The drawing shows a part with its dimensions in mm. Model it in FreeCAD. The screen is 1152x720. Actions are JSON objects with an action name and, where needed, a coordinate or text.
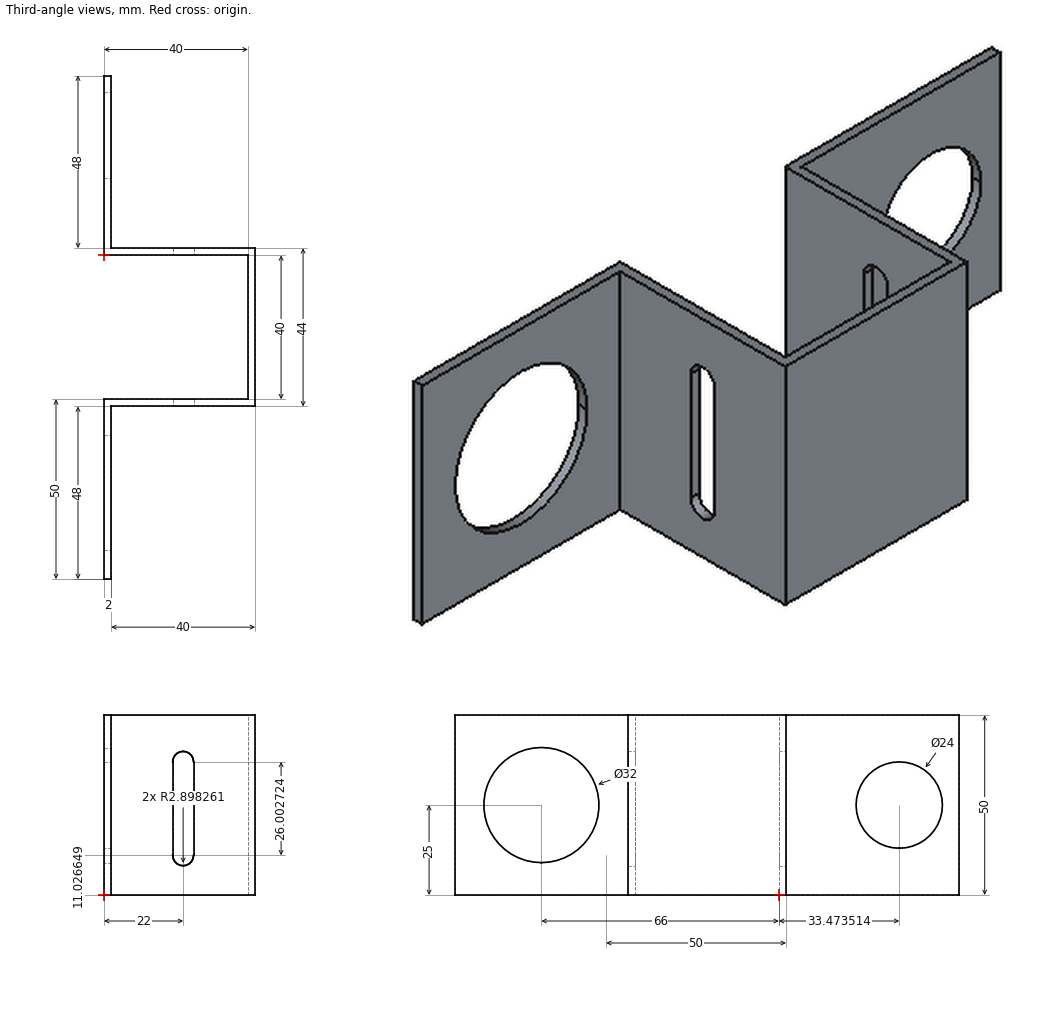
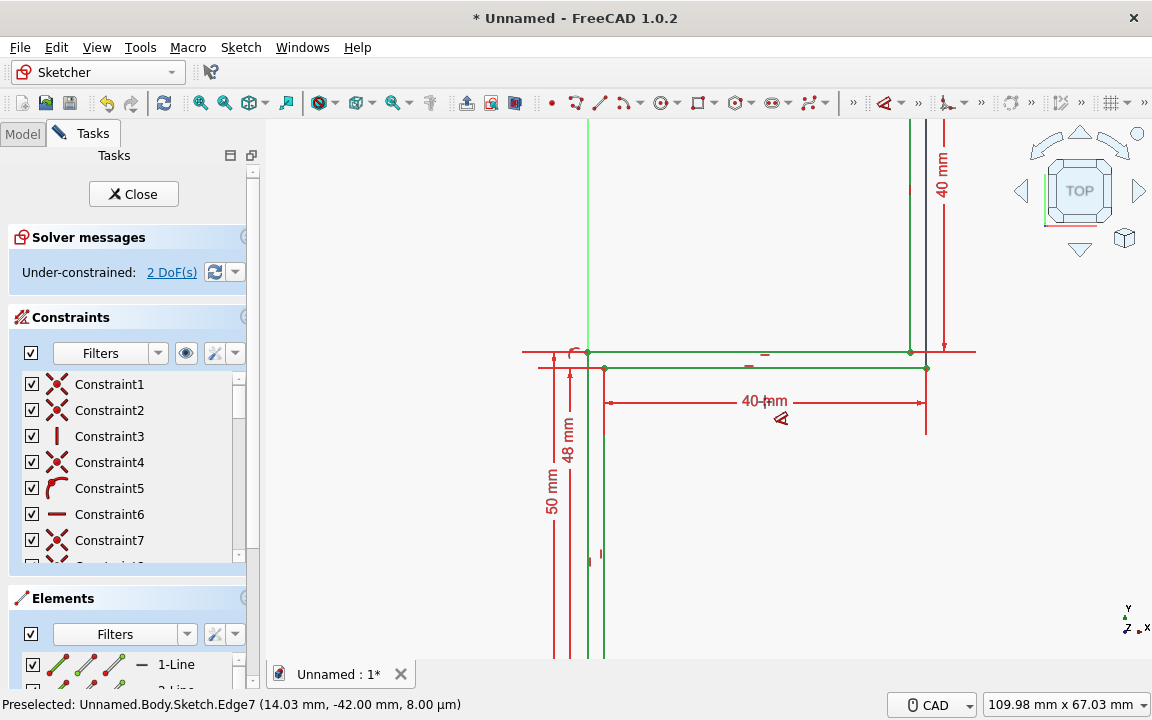
{"action": "left_click", "coordinate": [926, 262]}
{"action": "left_click", "coordinate": [960, 258]}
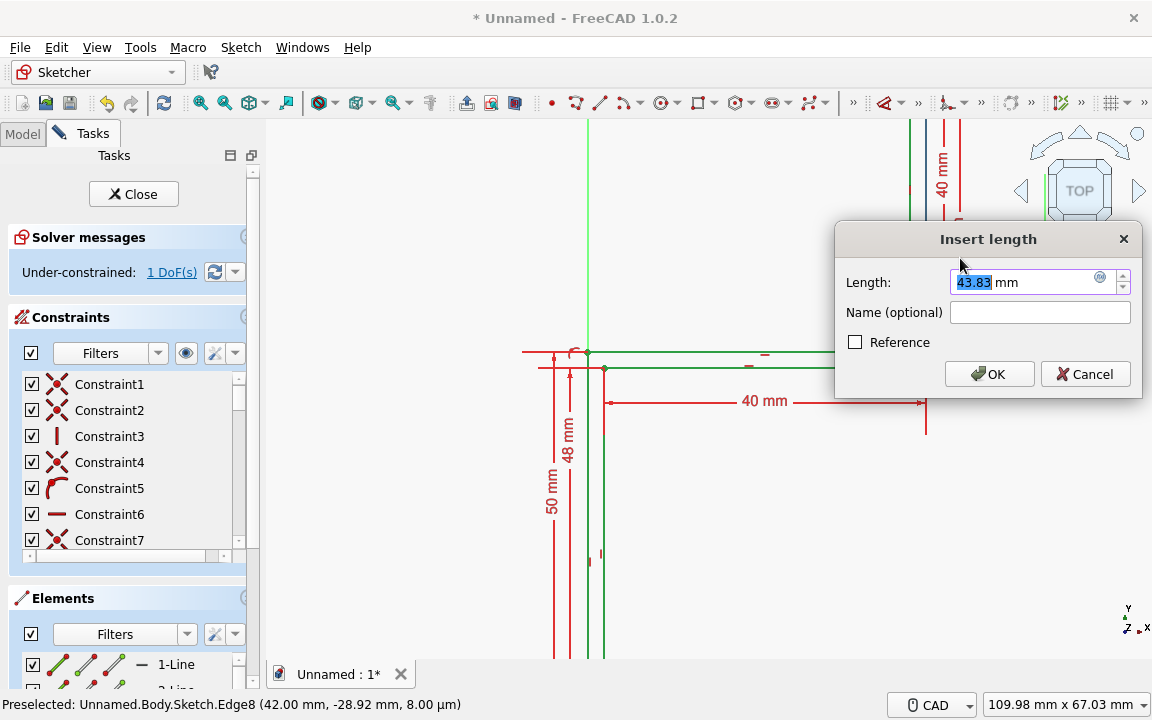
{"action": "type", "text": "44"}
{"action": "key", "text": "Return"}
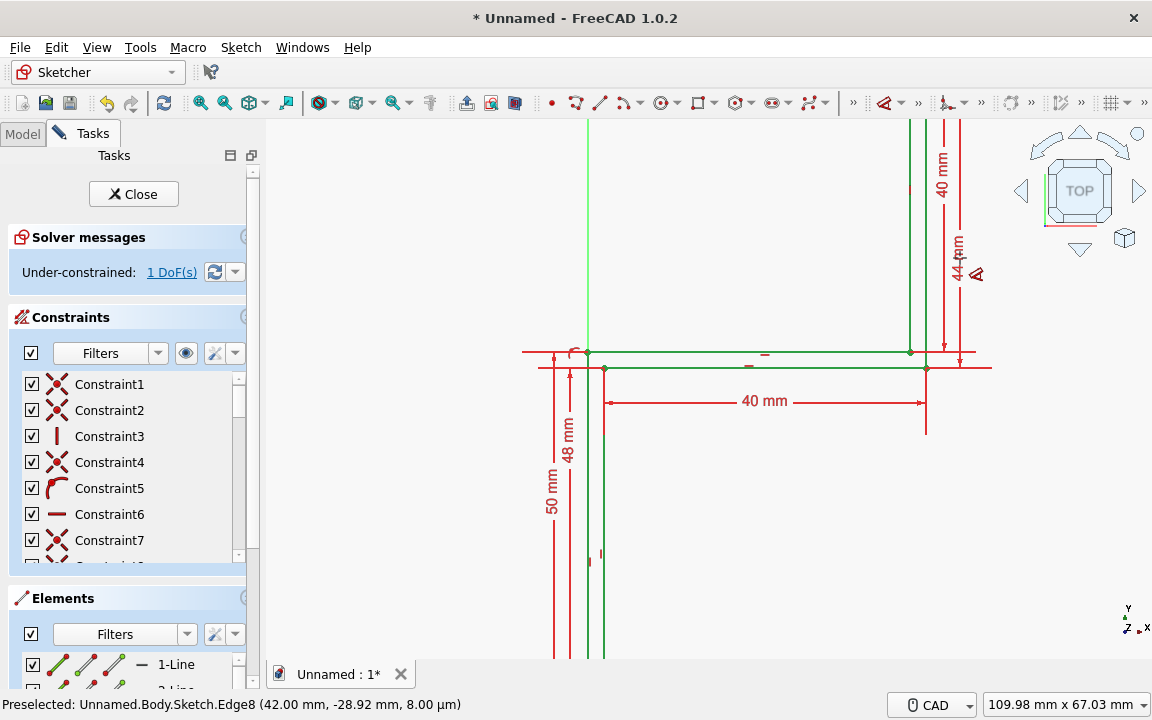
{"action": "scroll", "coordinate": [590, 474], "scroll_direction": "down", "scroll_amount": 6}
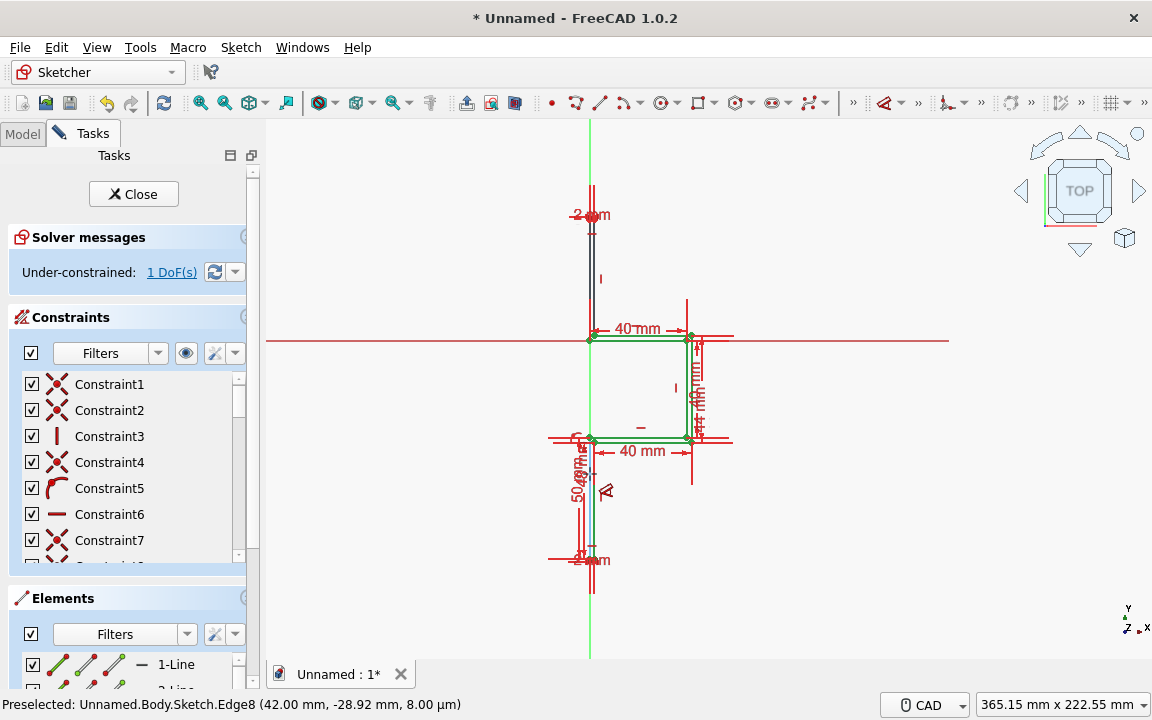
{"action": "scroll", "coordinate": [594, 301], "scroll_direction": "up", "scroll_amount": 6}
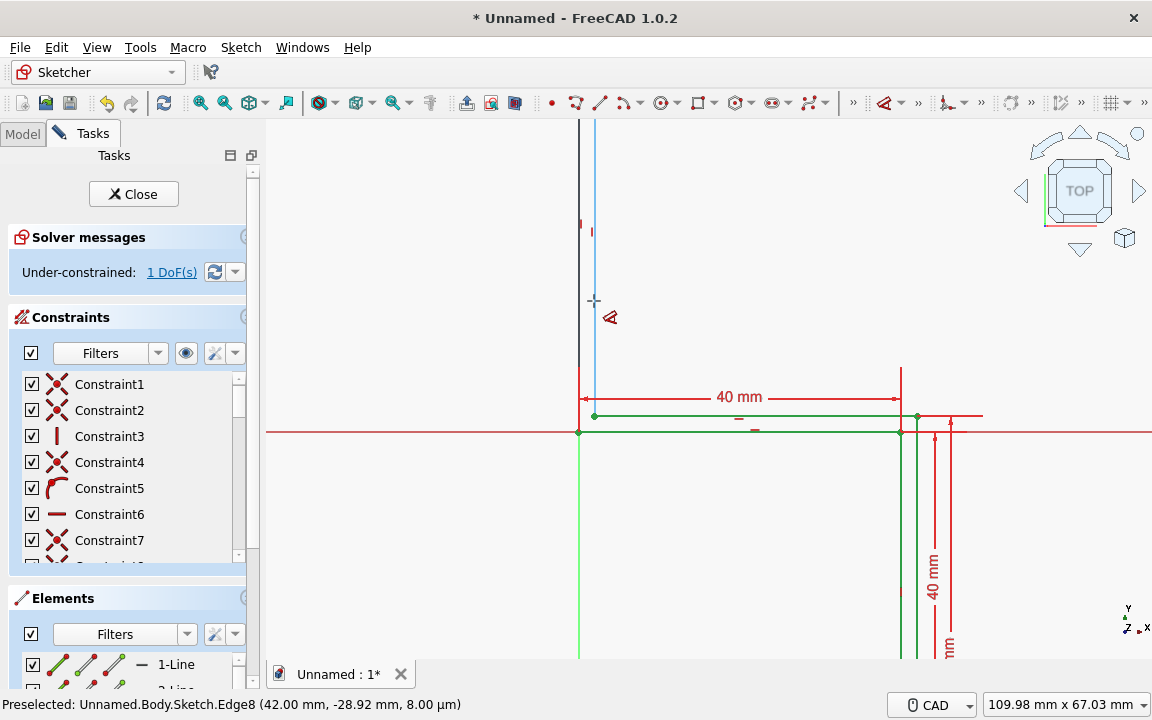
{"action": "left_click", "coordinate": [595, 300]}
{"action": "left_click", "coordinate": [561, 282]}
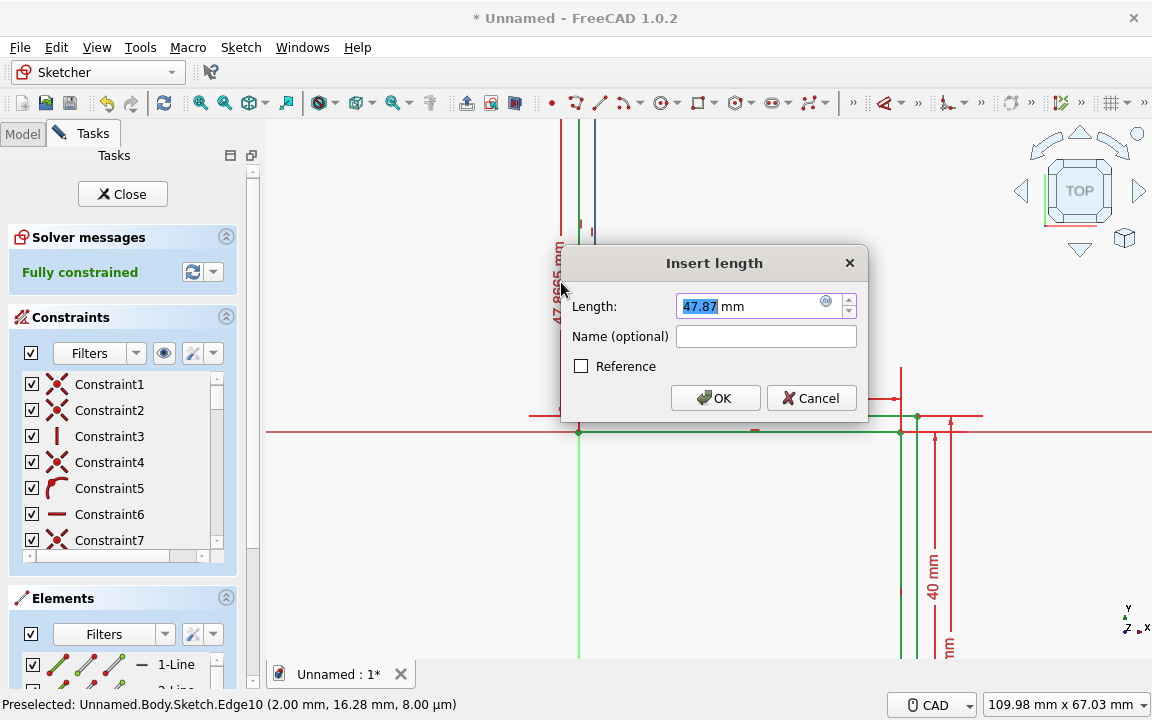
{"action": "type", "text": "48"}
{"action": "key", "text": "Return"}
{"action": "key", "text": "Escape"}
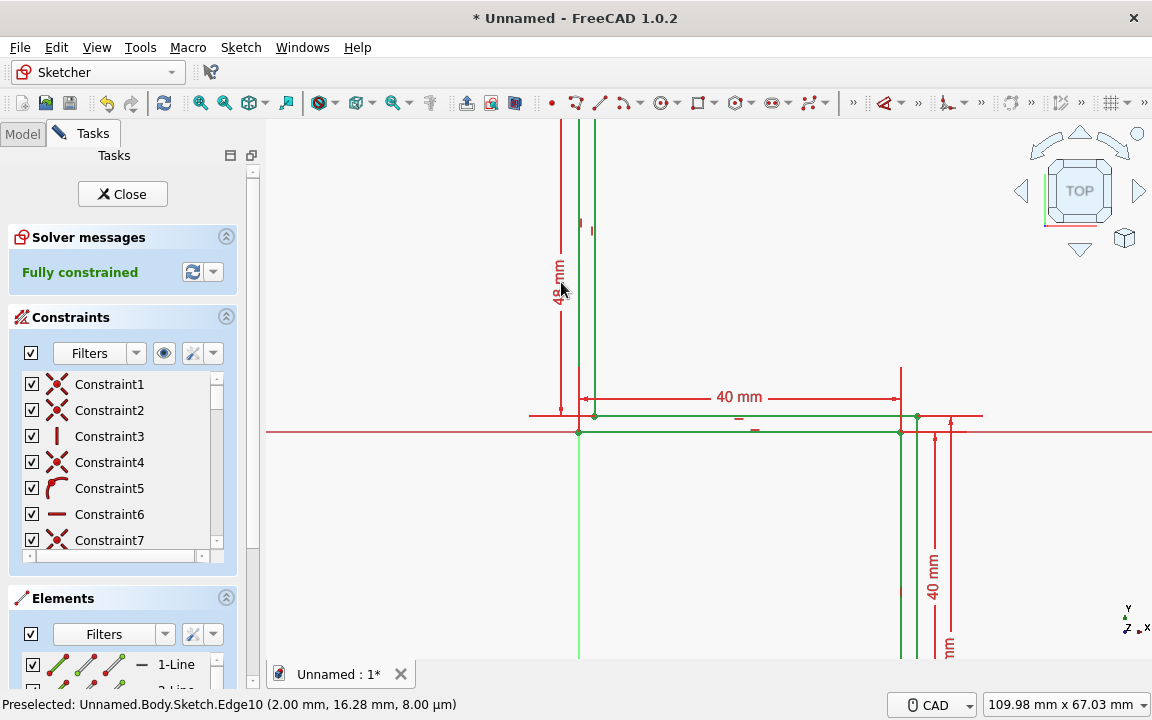
{"action": "left_click", "coordinate": [123, 194]}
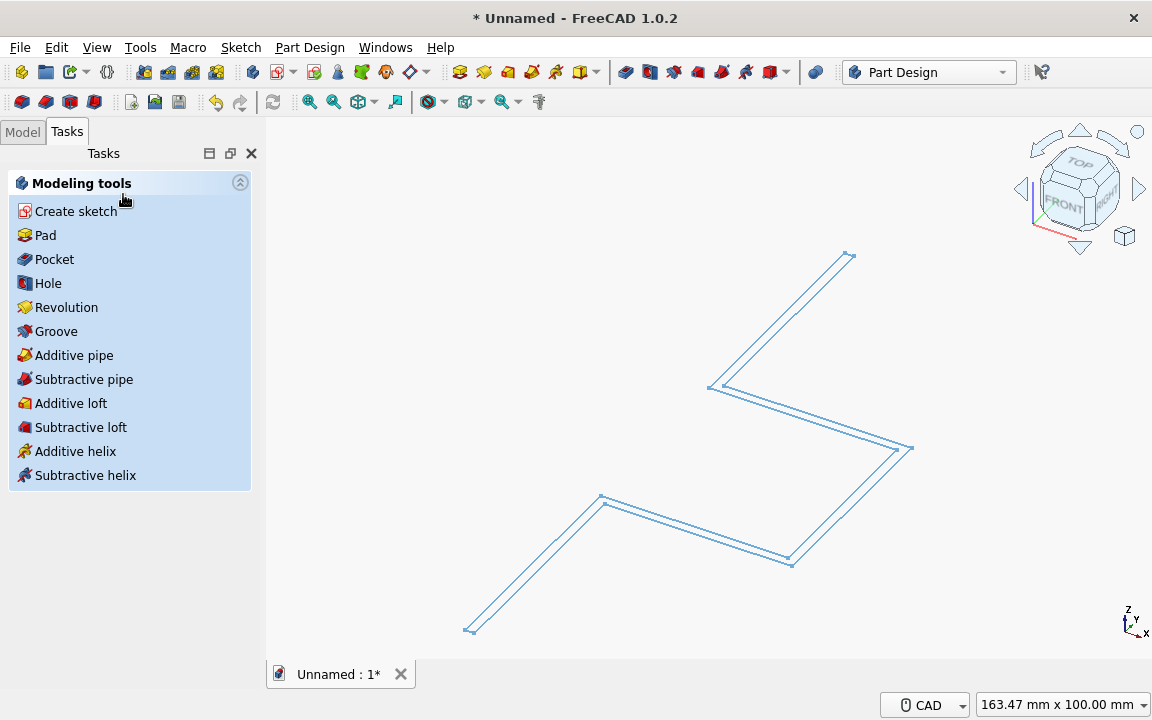
{"action": "left_click", "coordinate": [460, 72]}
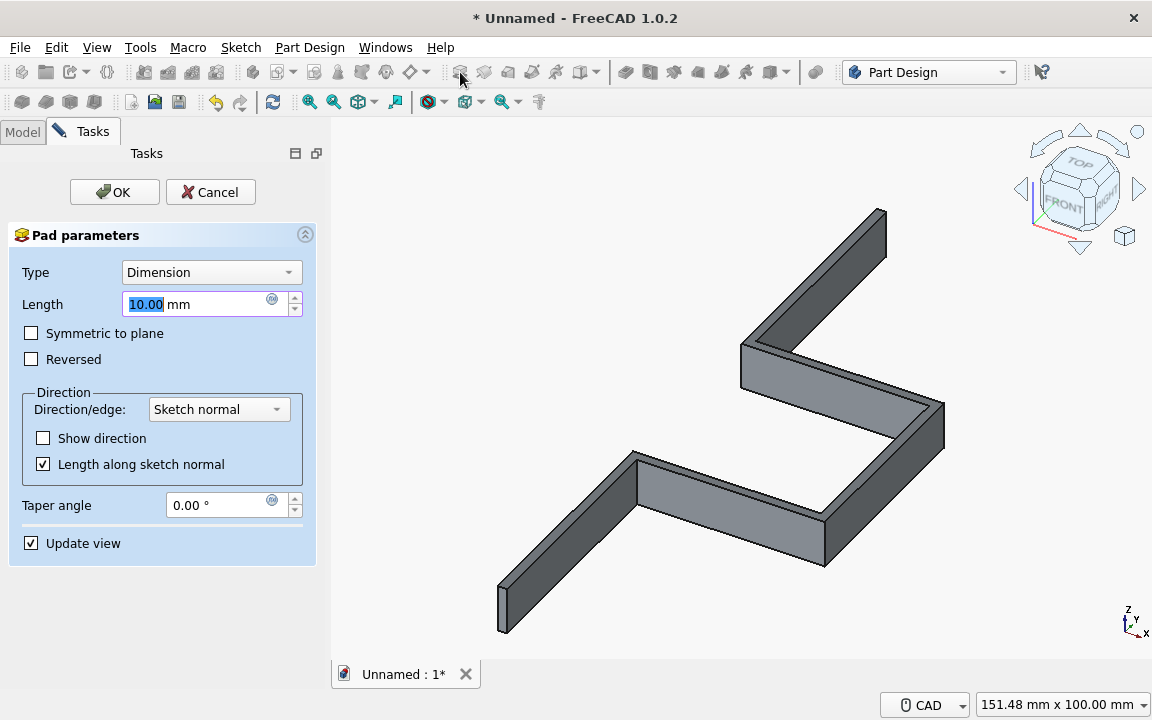
{"action": "type", "text": "50"}
{"action": "key", "text": "Tab"}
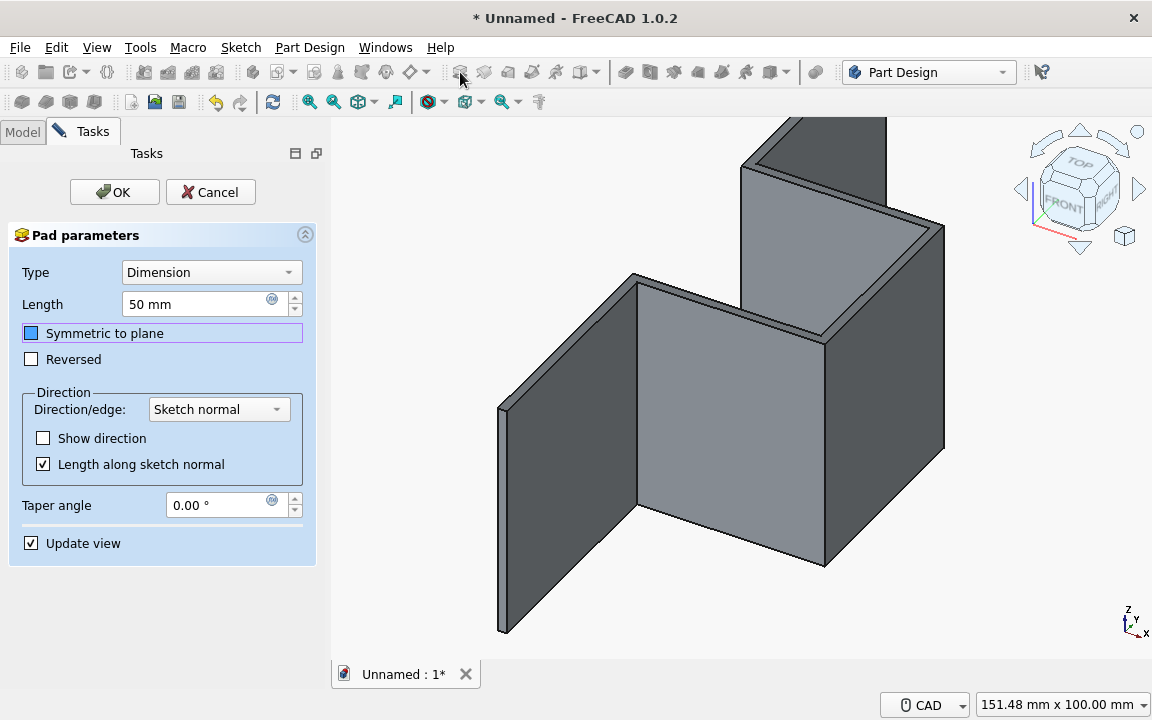
{"action": "left_click", "coordinate": [115, 192]}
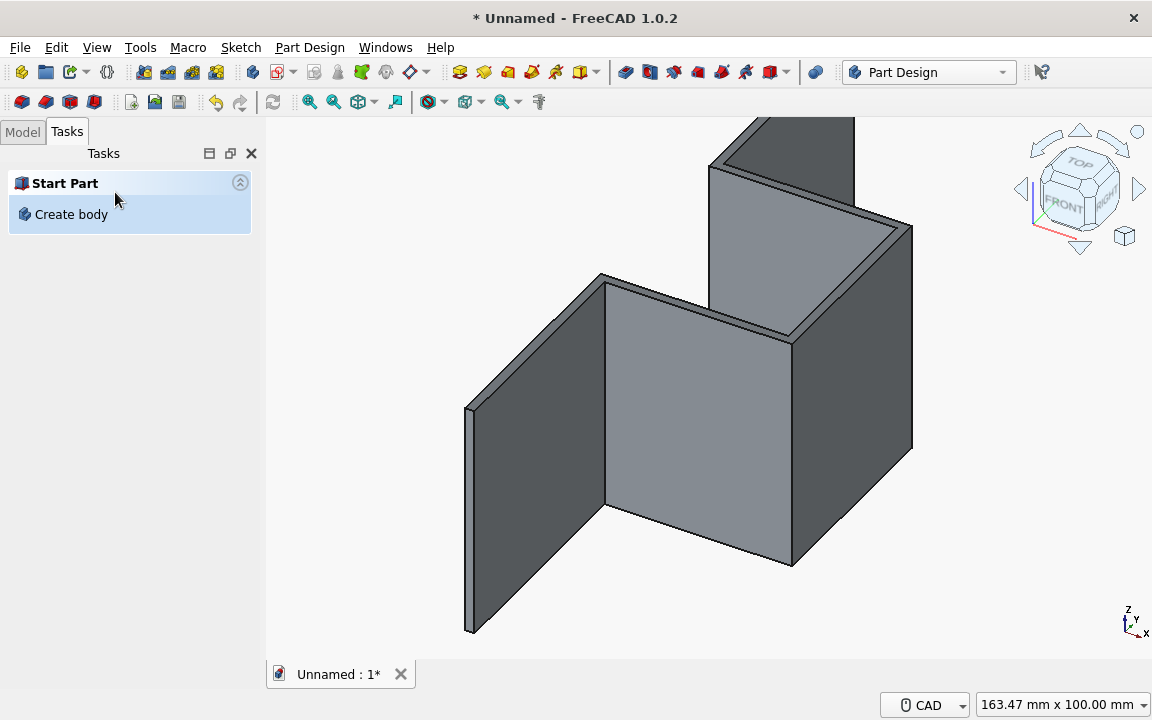
{"action": "left_click", "coordinate": [310, 102]}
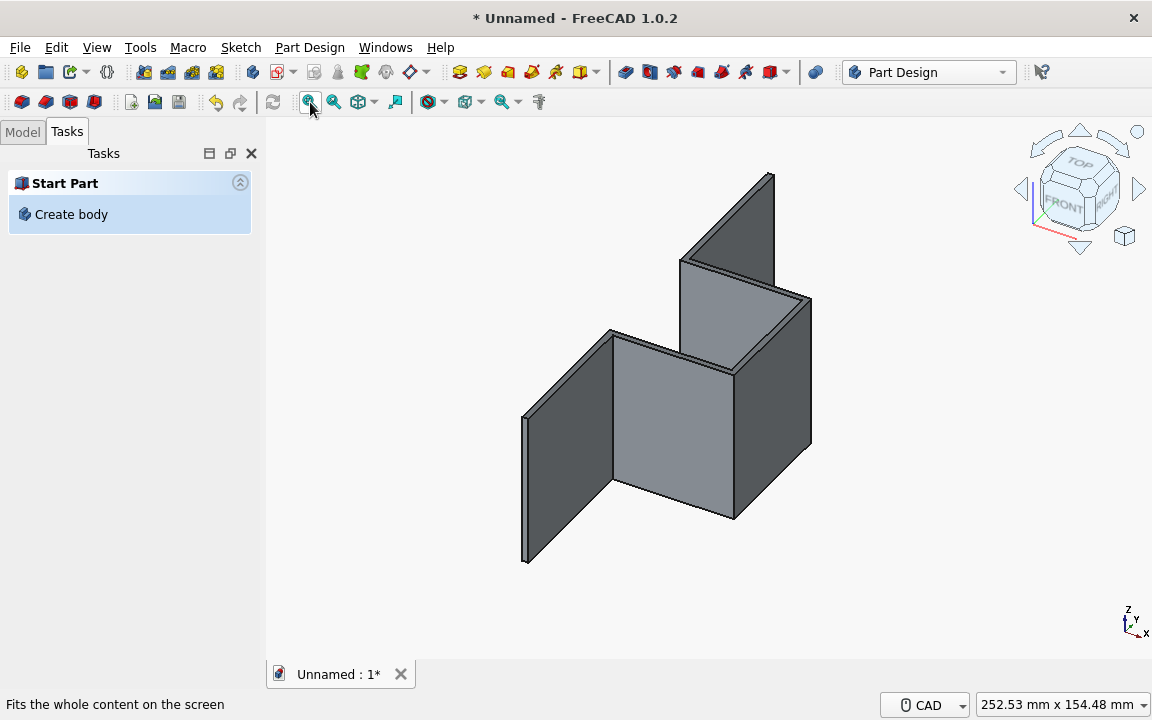
{"action": "key", "text": "4"}